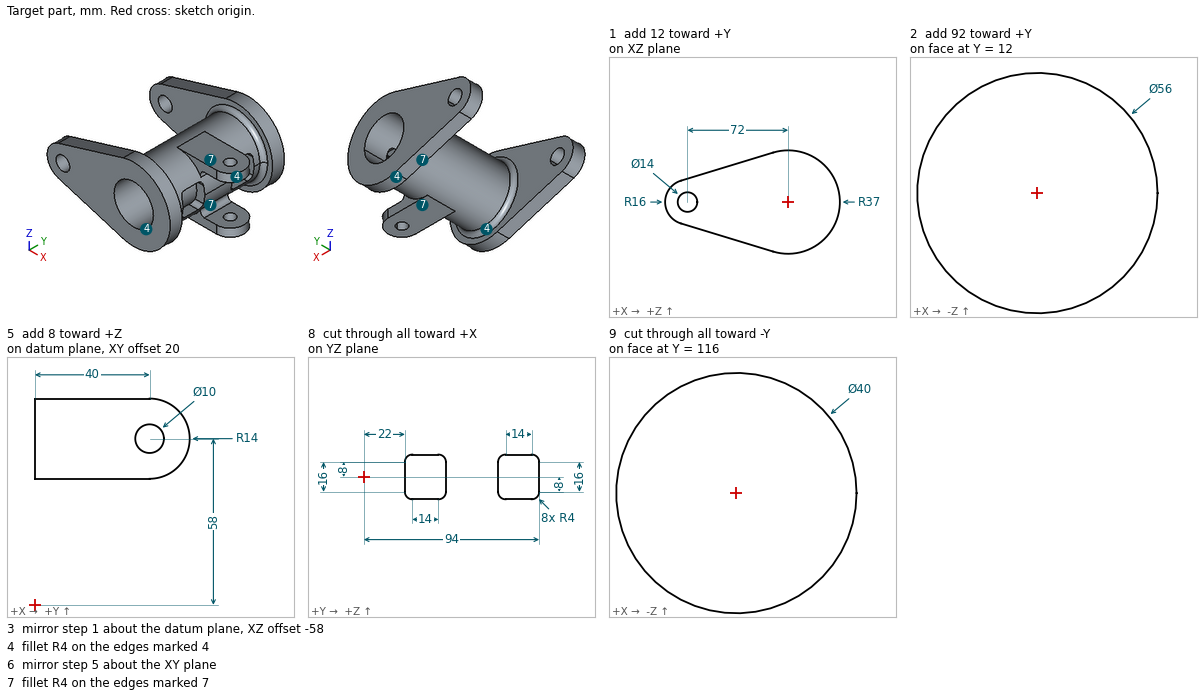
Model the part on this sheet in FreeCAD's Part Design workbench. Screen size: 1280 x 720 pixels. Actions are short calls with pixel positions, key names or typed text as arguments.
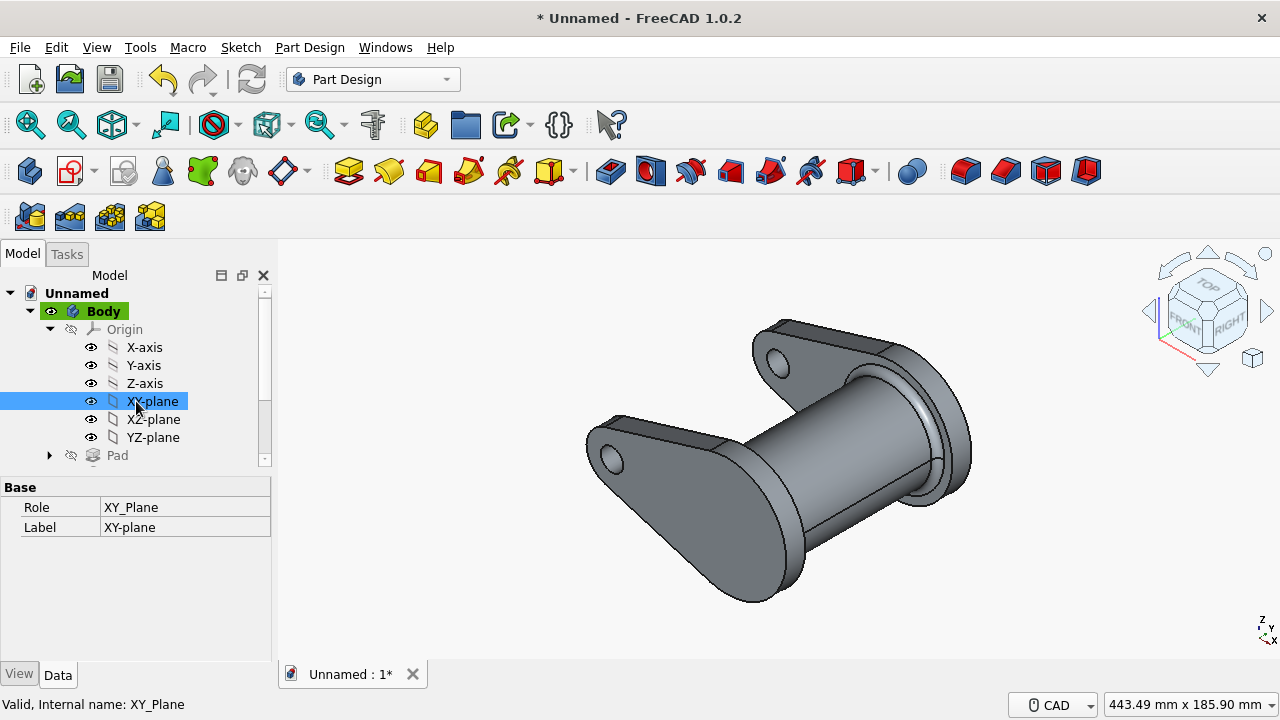
click(284, 172)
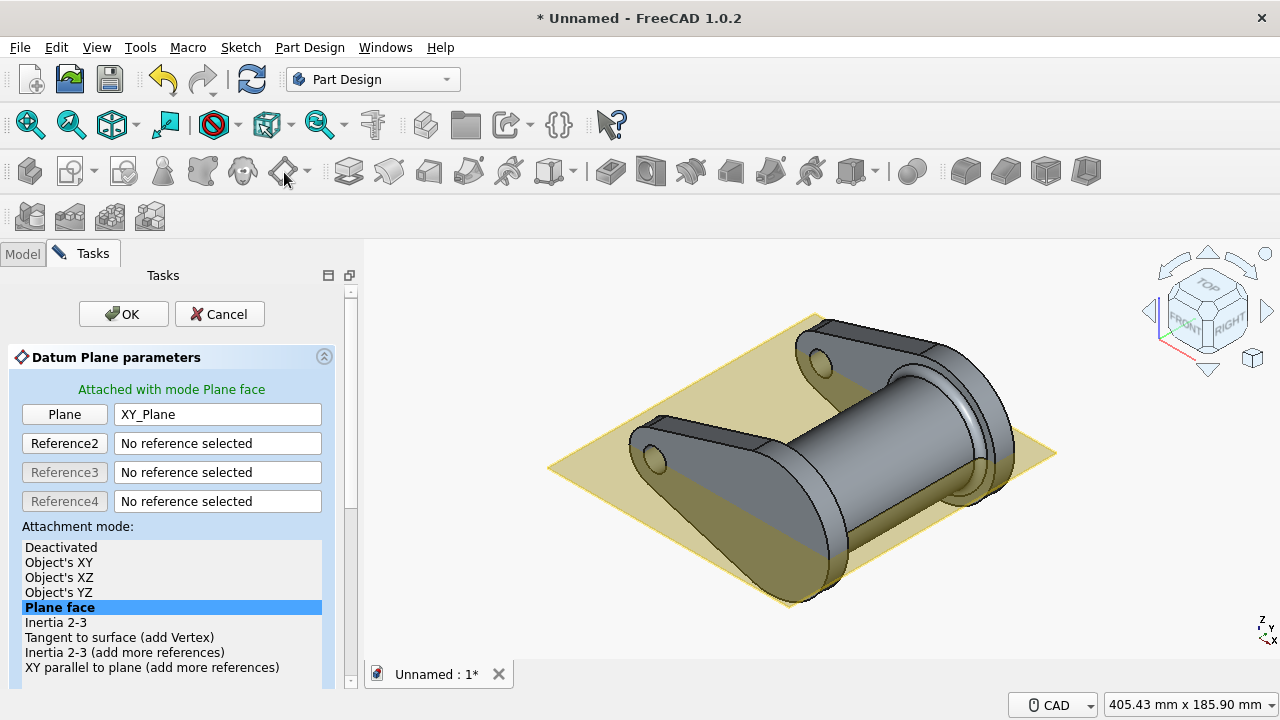
scroll(351, 486, down, 4)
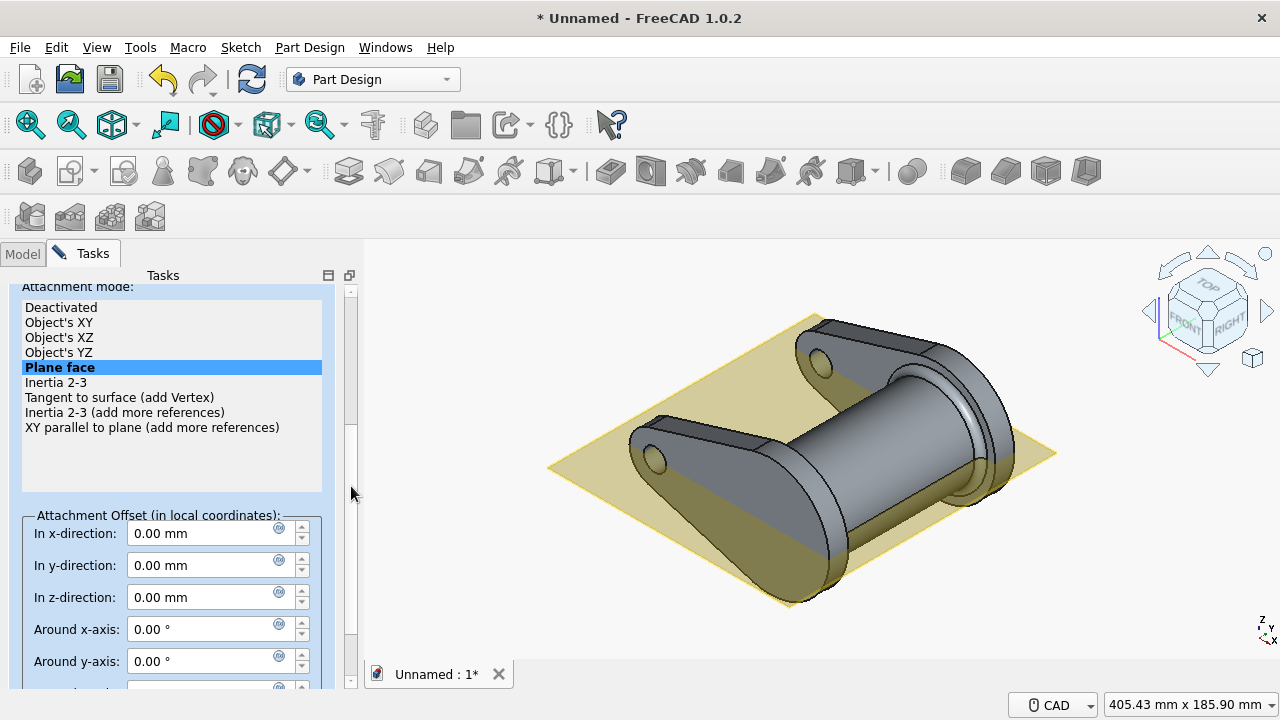
triple_click(210, 597)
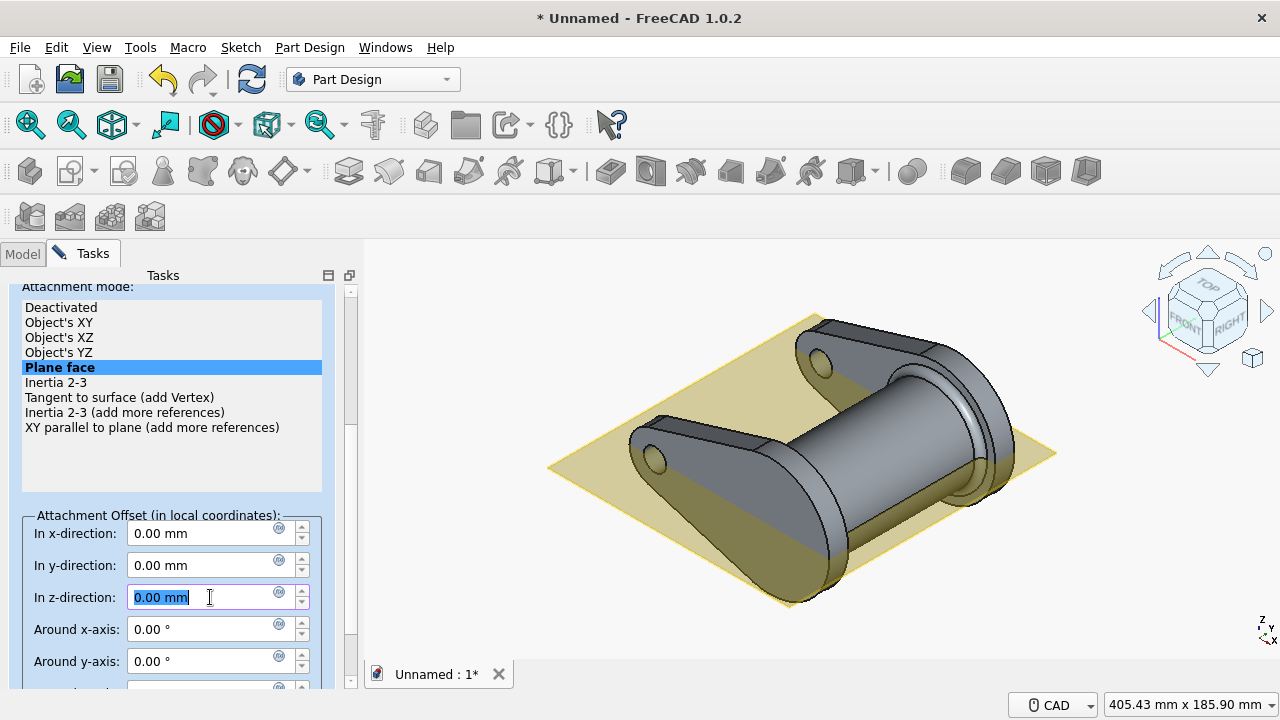
text(20)
key(Tab)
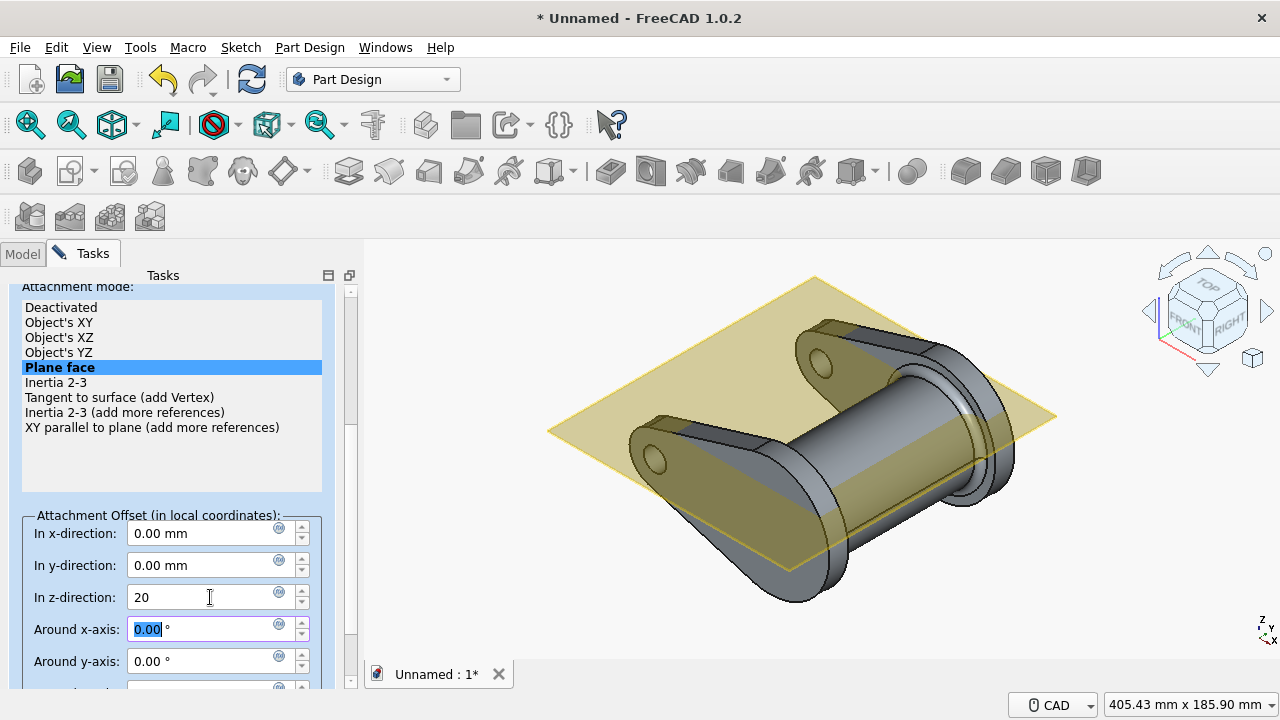
scroll(351, 486, up, 5)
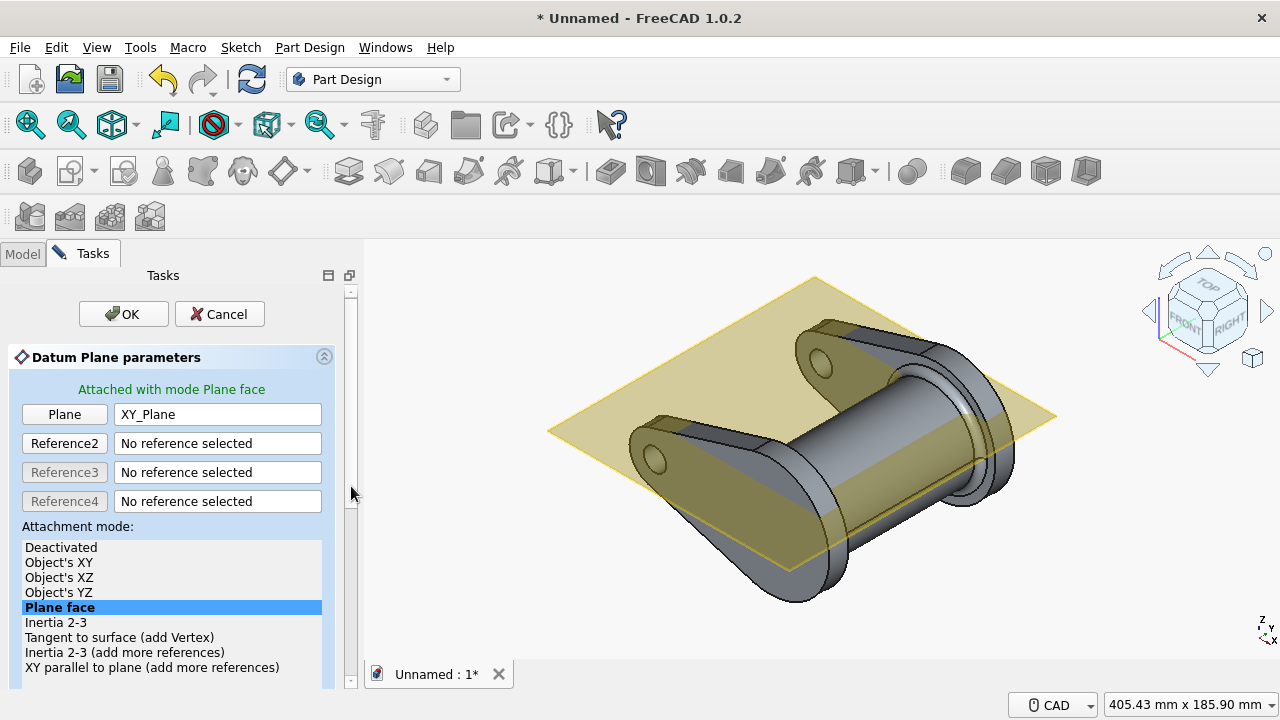
click(124, 314)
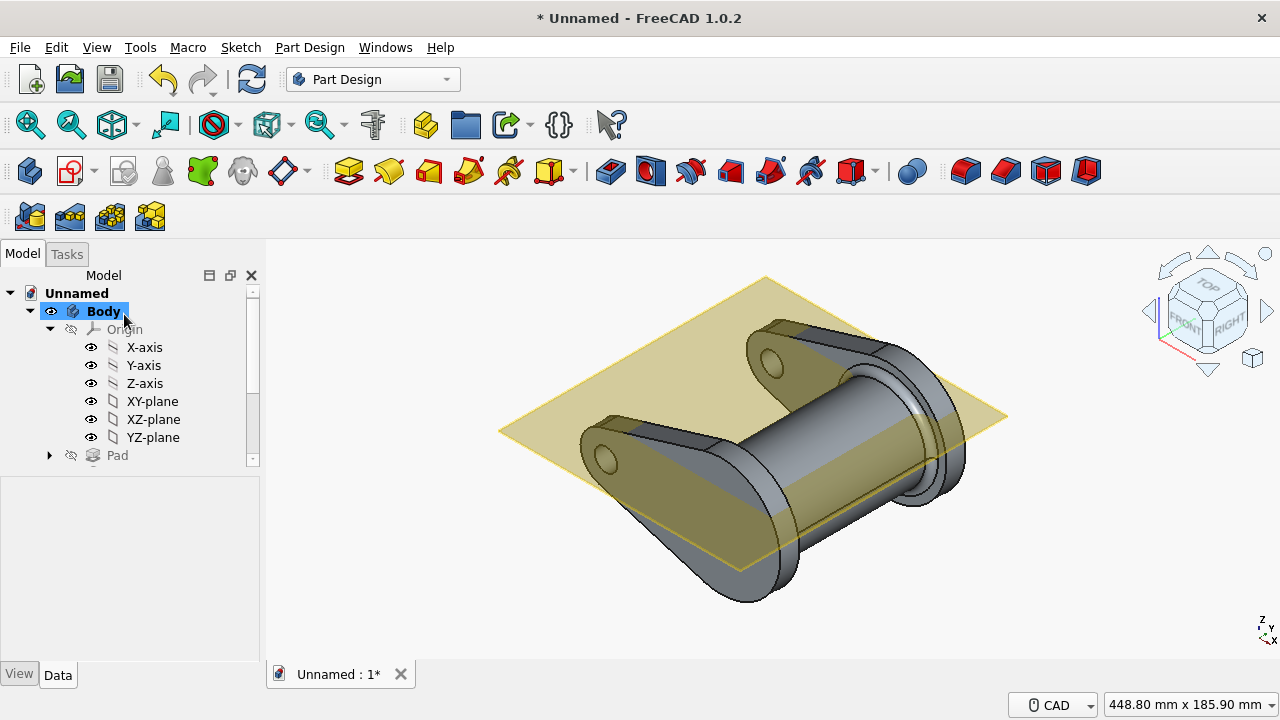
scroll(100, 379, down, 3)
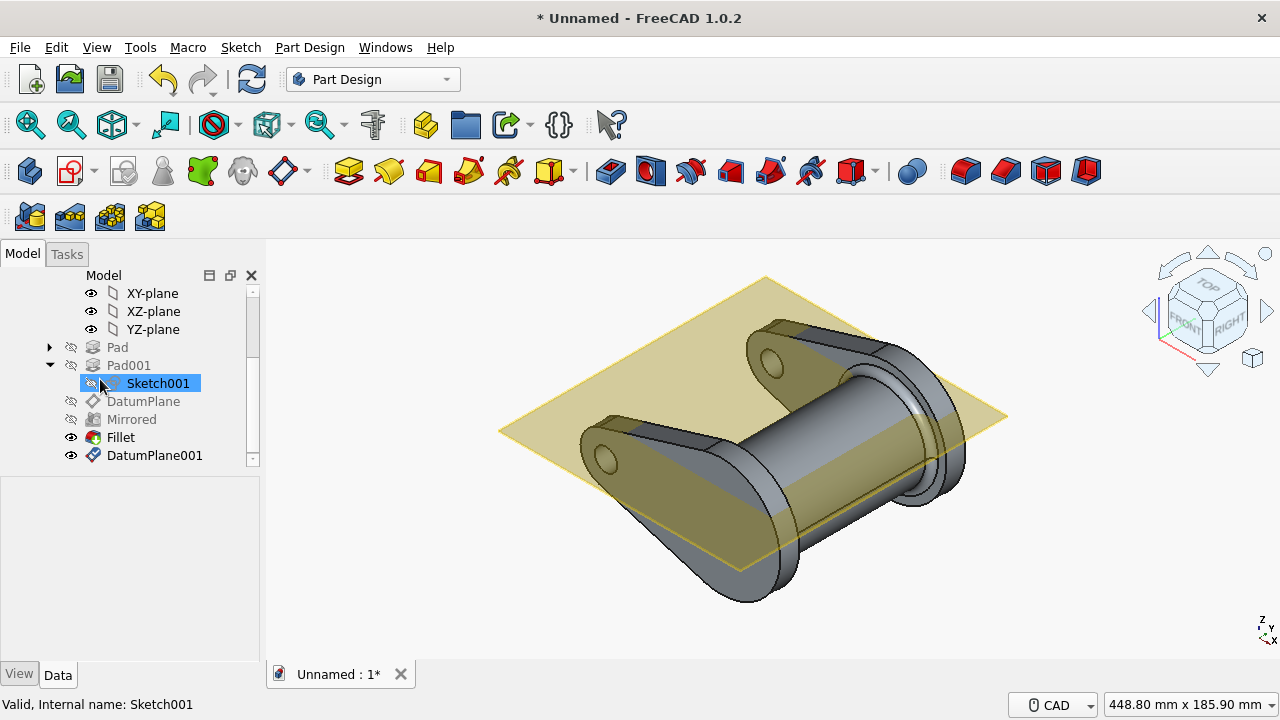
click(116, 455)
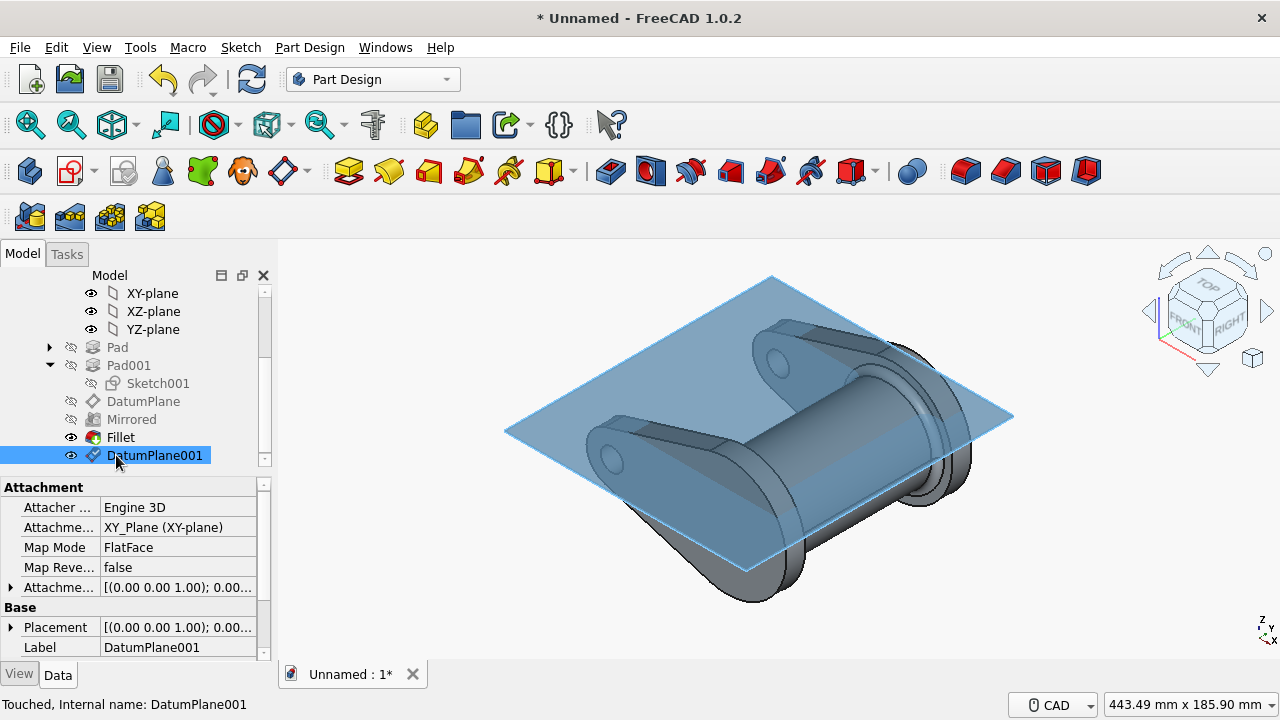
click(70, 172)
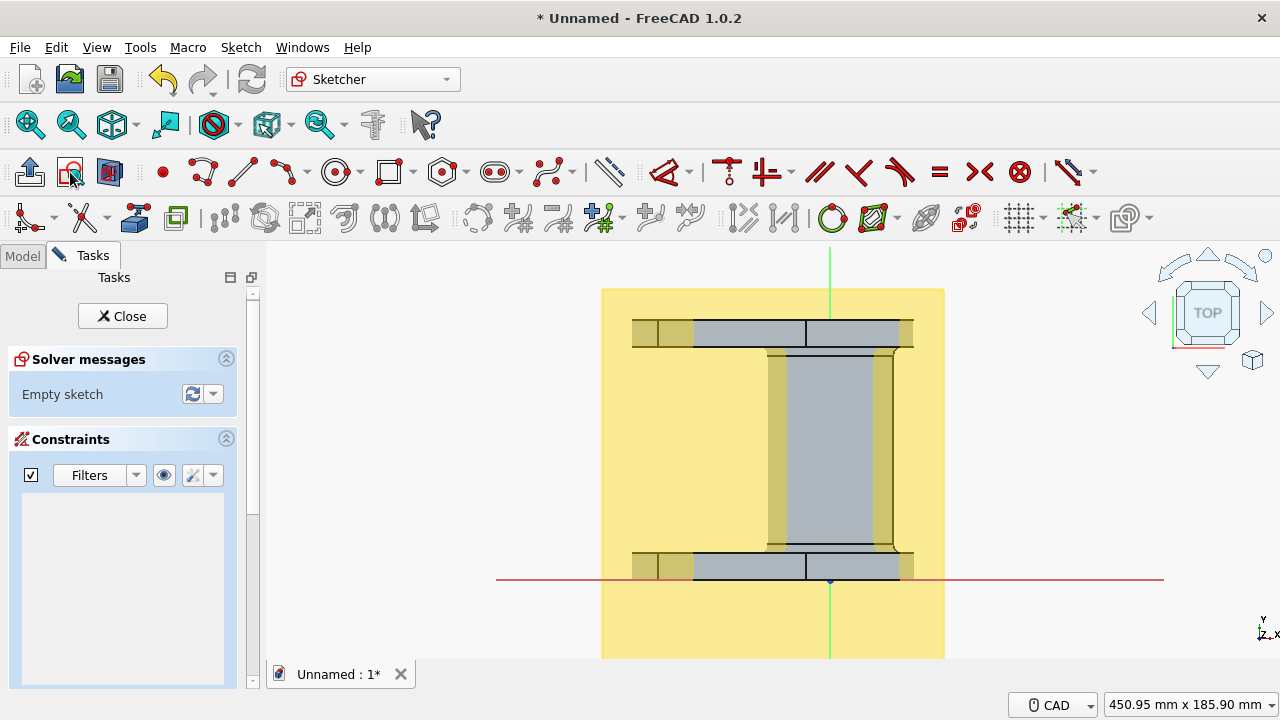
click(110, 172)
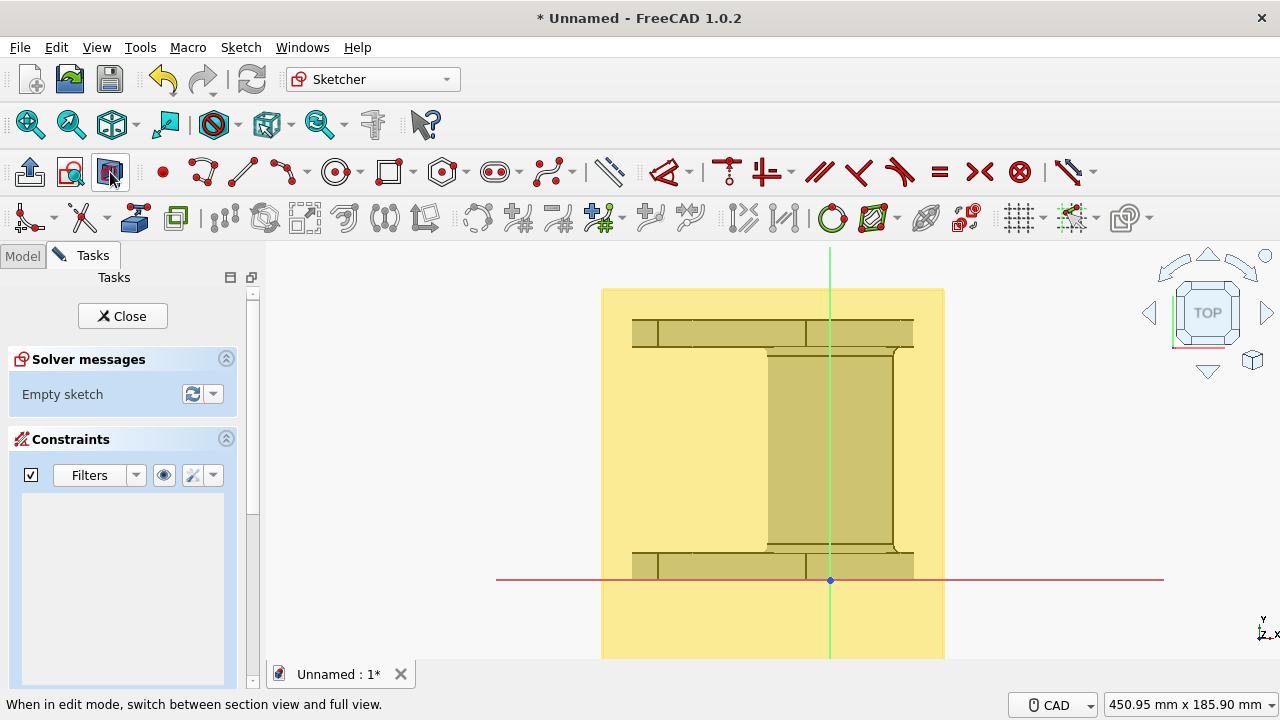
scroll(1115, 600, up, 2)